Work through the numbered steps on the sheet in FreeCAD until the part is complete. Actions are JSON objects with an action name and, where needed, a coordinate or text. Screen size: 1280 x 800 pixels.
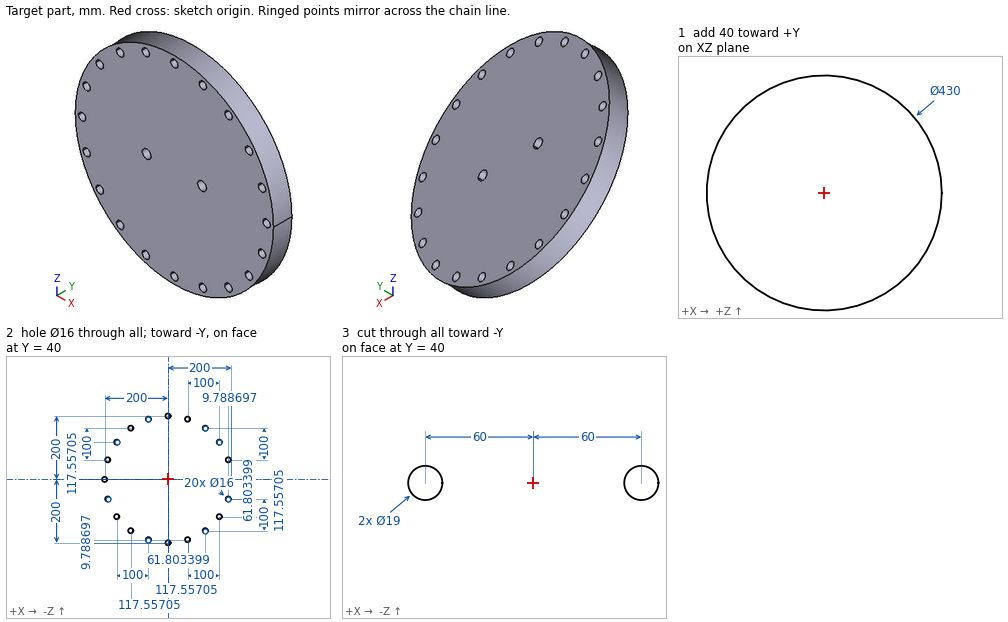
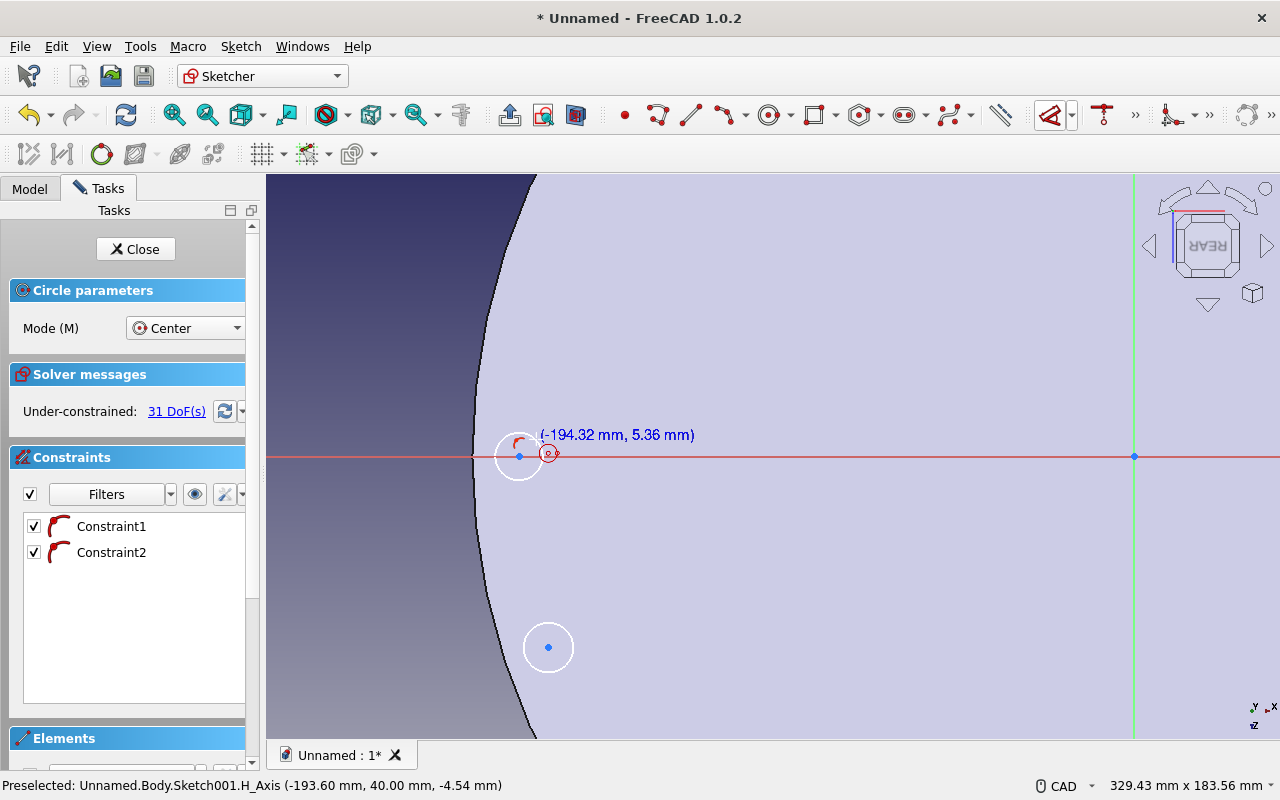
{"action": "left_click", "coordinate": [549, 266]}
{"action": "left_click", "coordinate": [566, 249]}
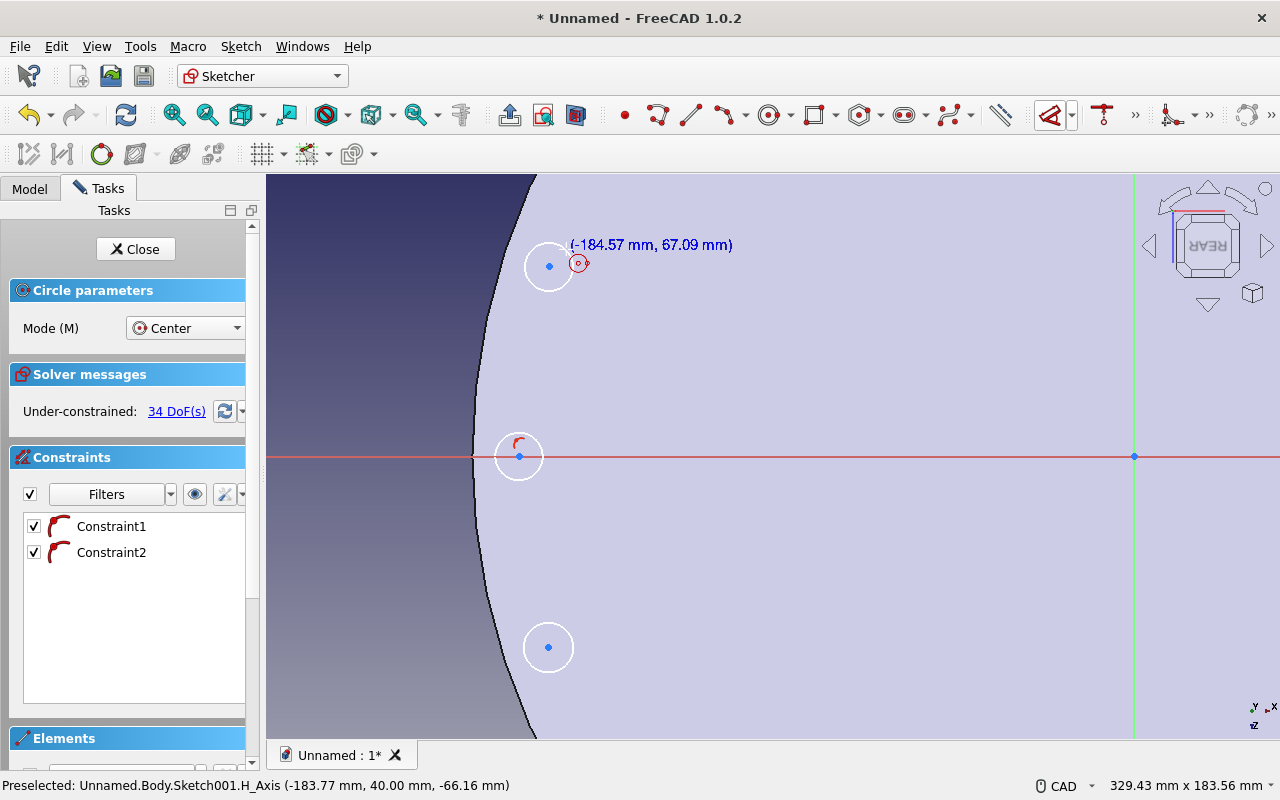
{"action": "scroll", "coordinate": [519, 456], "scroll_direction": "down", "scroll_amount": 6}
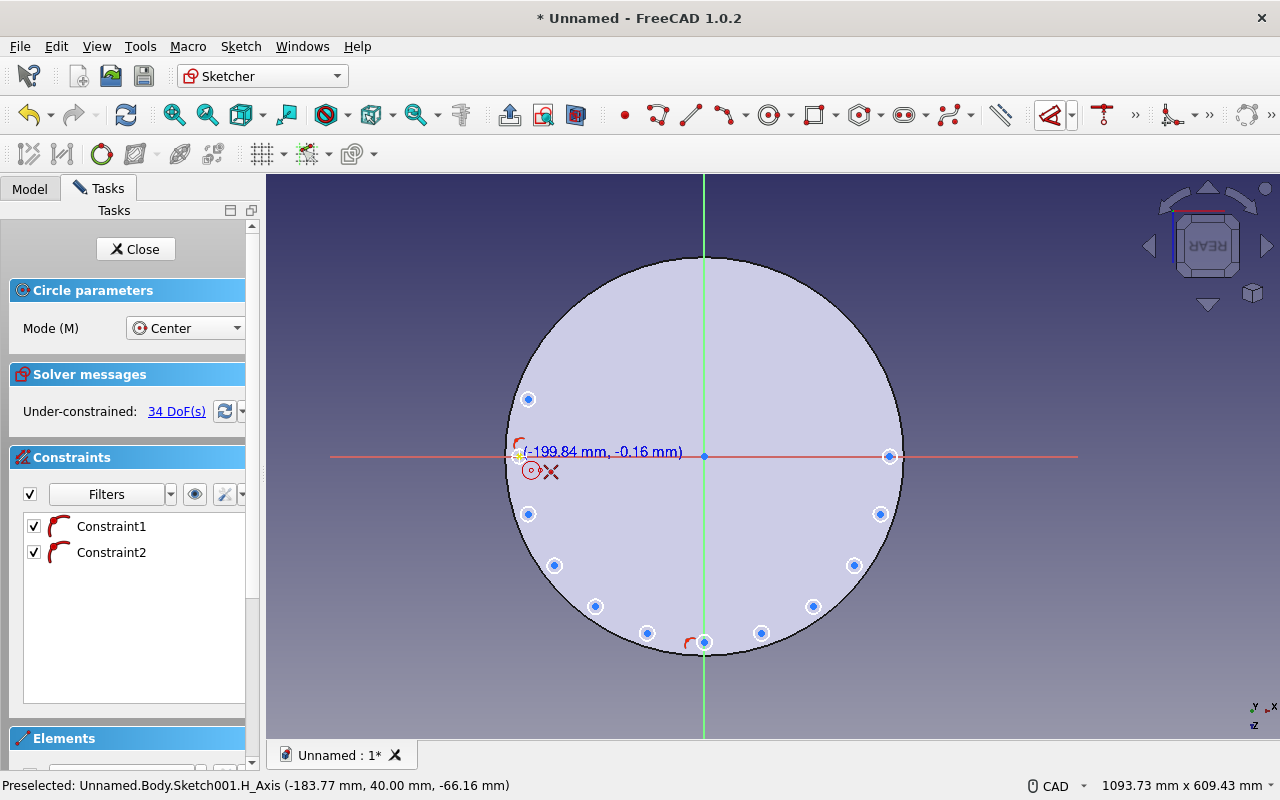
{"action": "scroll", "coordinate": [554, 348], "scroll_direction": "up", "scroll_amount": 6}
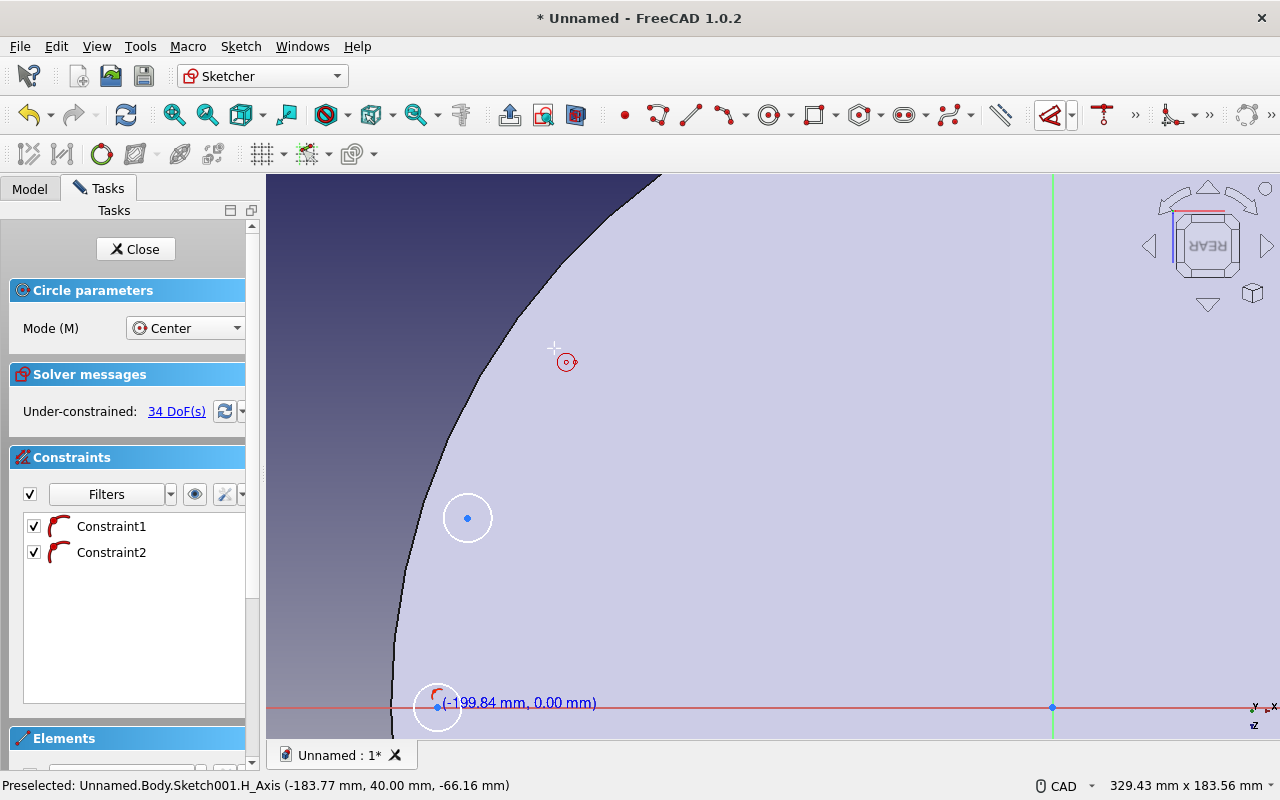
{"action": "left_click", "coordinate": [555, 346]}
{"action": "left_click", "coordinate": [572, 328]}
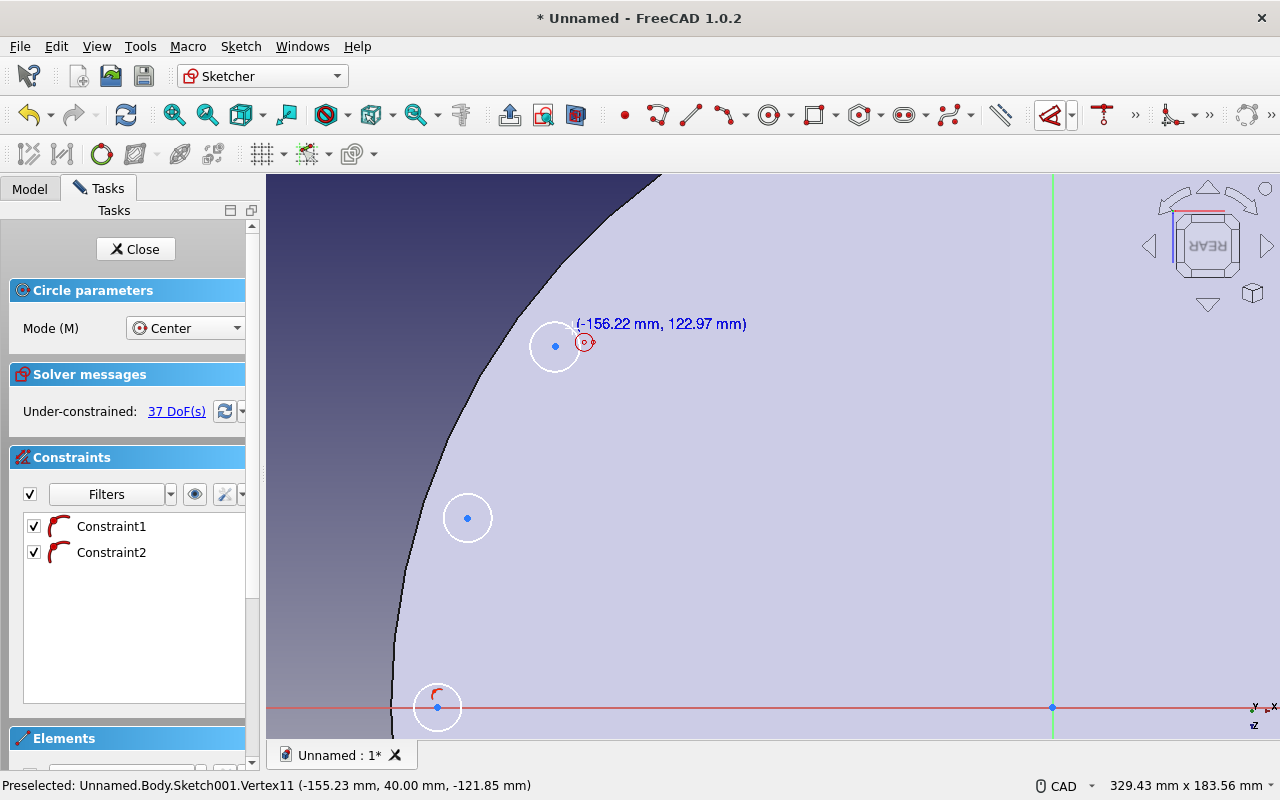
{"action": "left_click", "coordinate": [691, 209]}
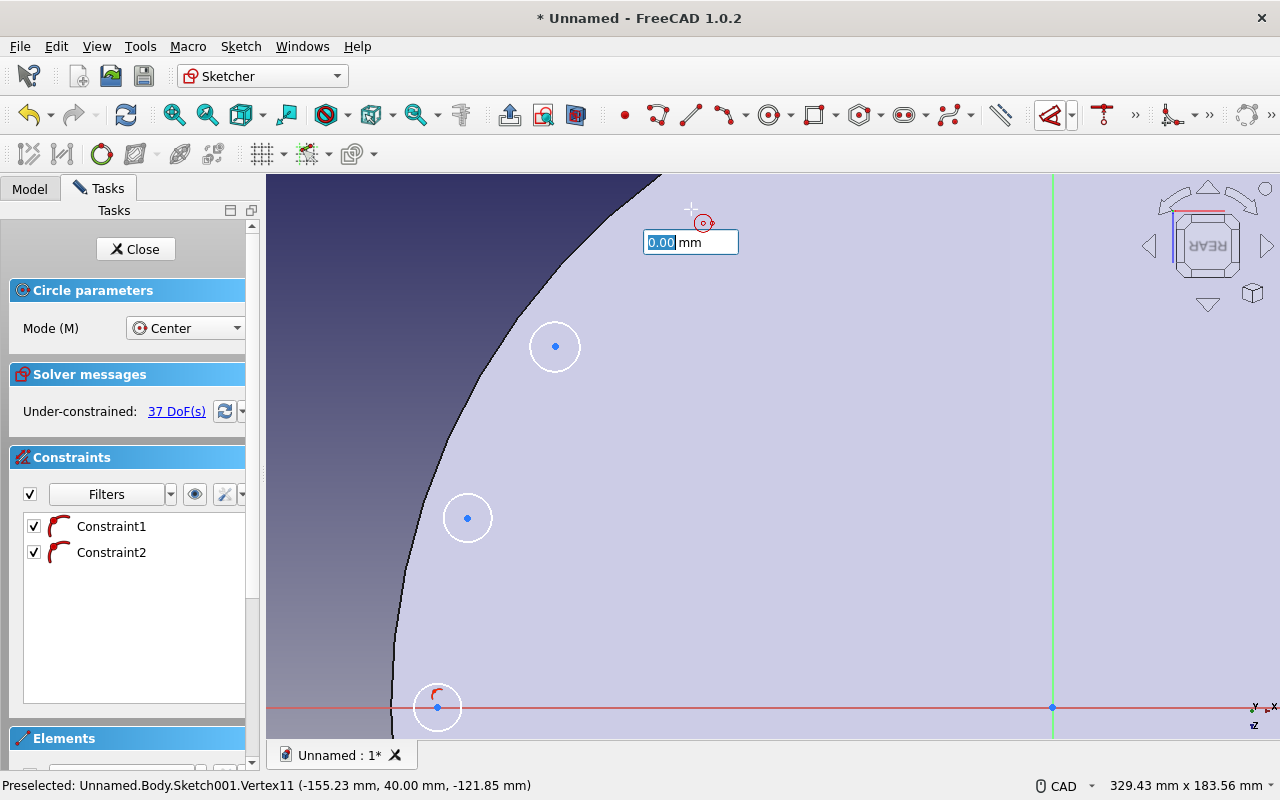
{"action": "scroll", "coordinate": [554, 348], "scroll_direction": "down", "scroll_amount": 6}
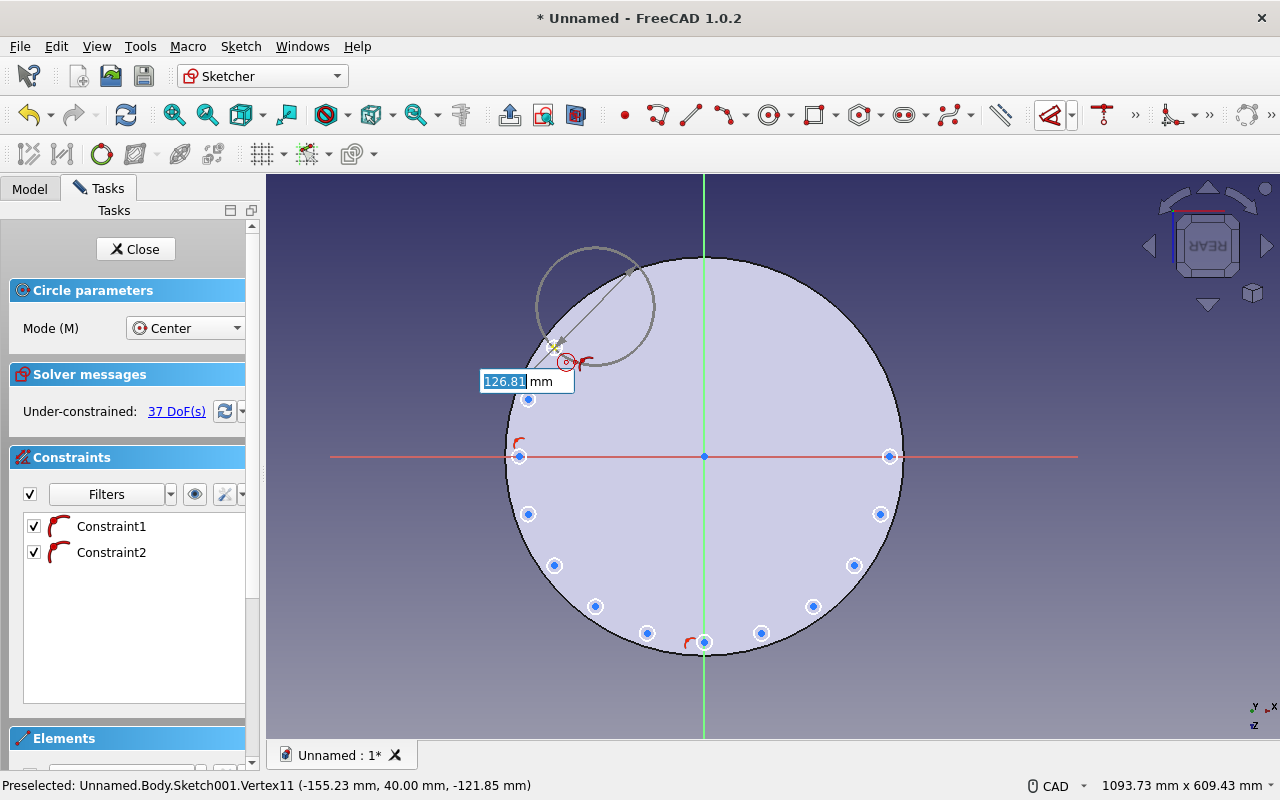
{"action": "scroll", "coordinate": [601, 301], "scroll_direction": "up", "scroll_amount": 4}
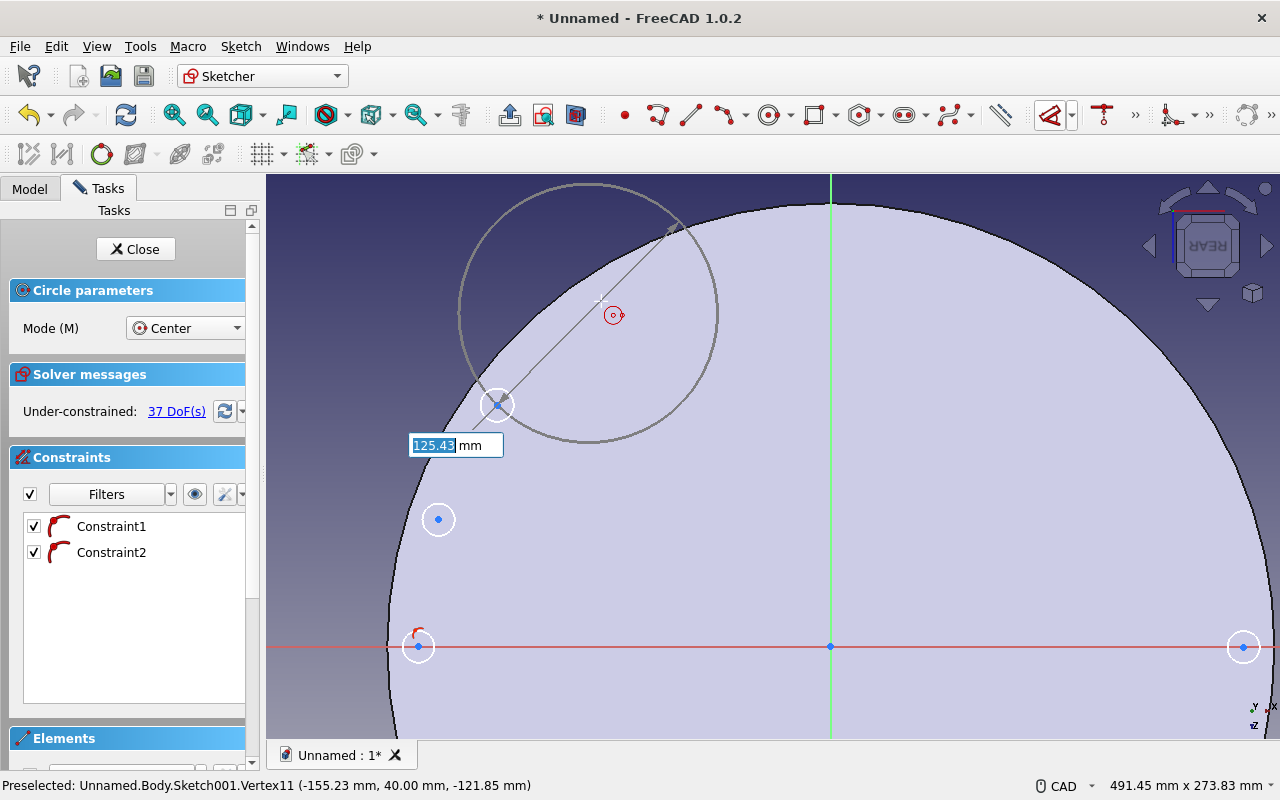
{"action": "left_click", "coordinate": [600, 301]}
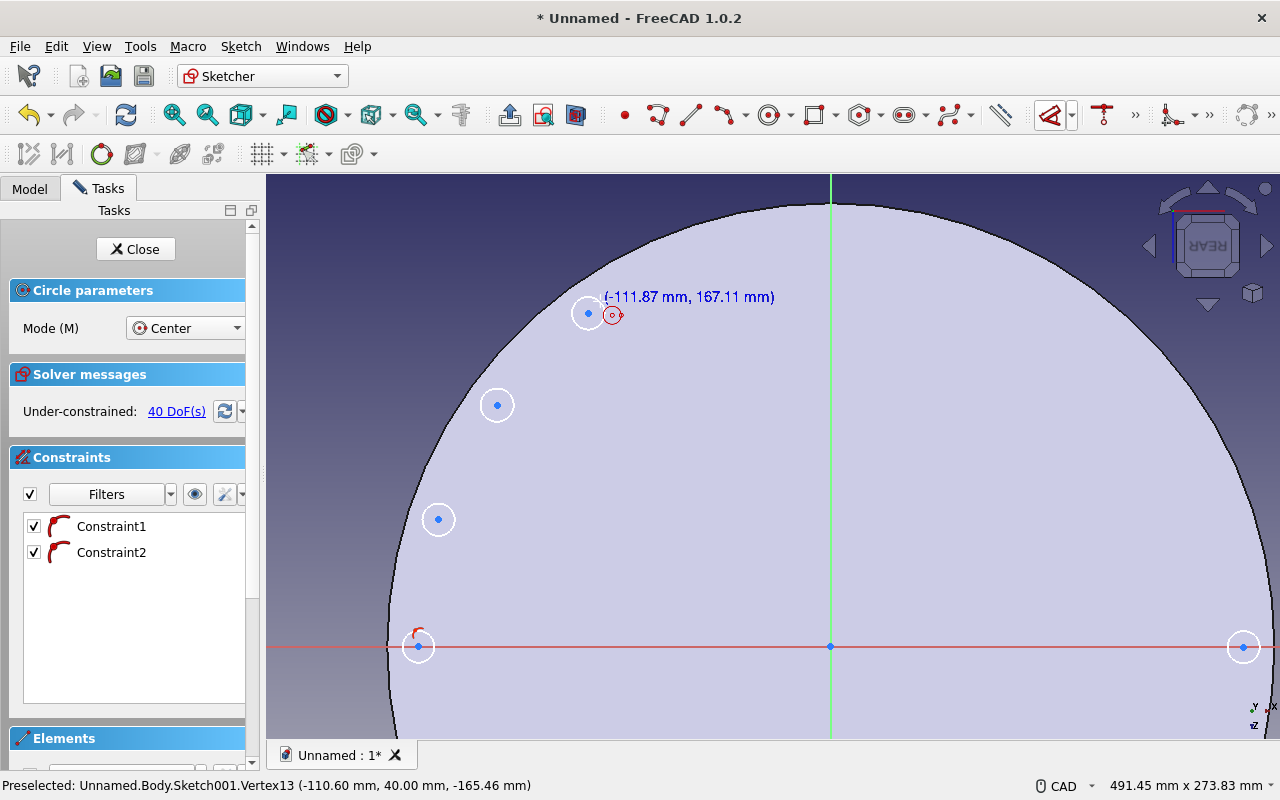
{"action": "scroll", "coordinate": [703, 254], "scroll_direction": "up", "scroll_amount": 2}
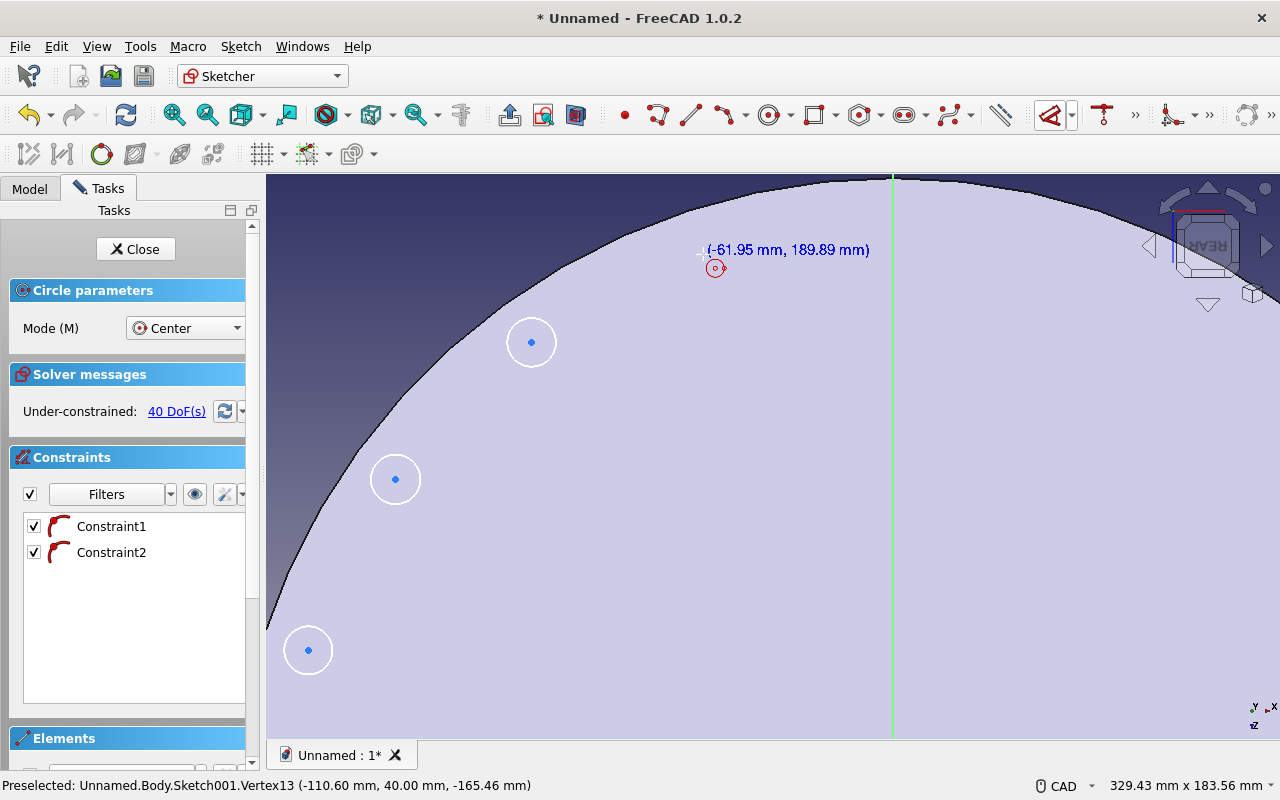
{"action": "left_click", "coordinate": [703, 254]}
{"action": "left_click", "coordinate": [721, 237]}